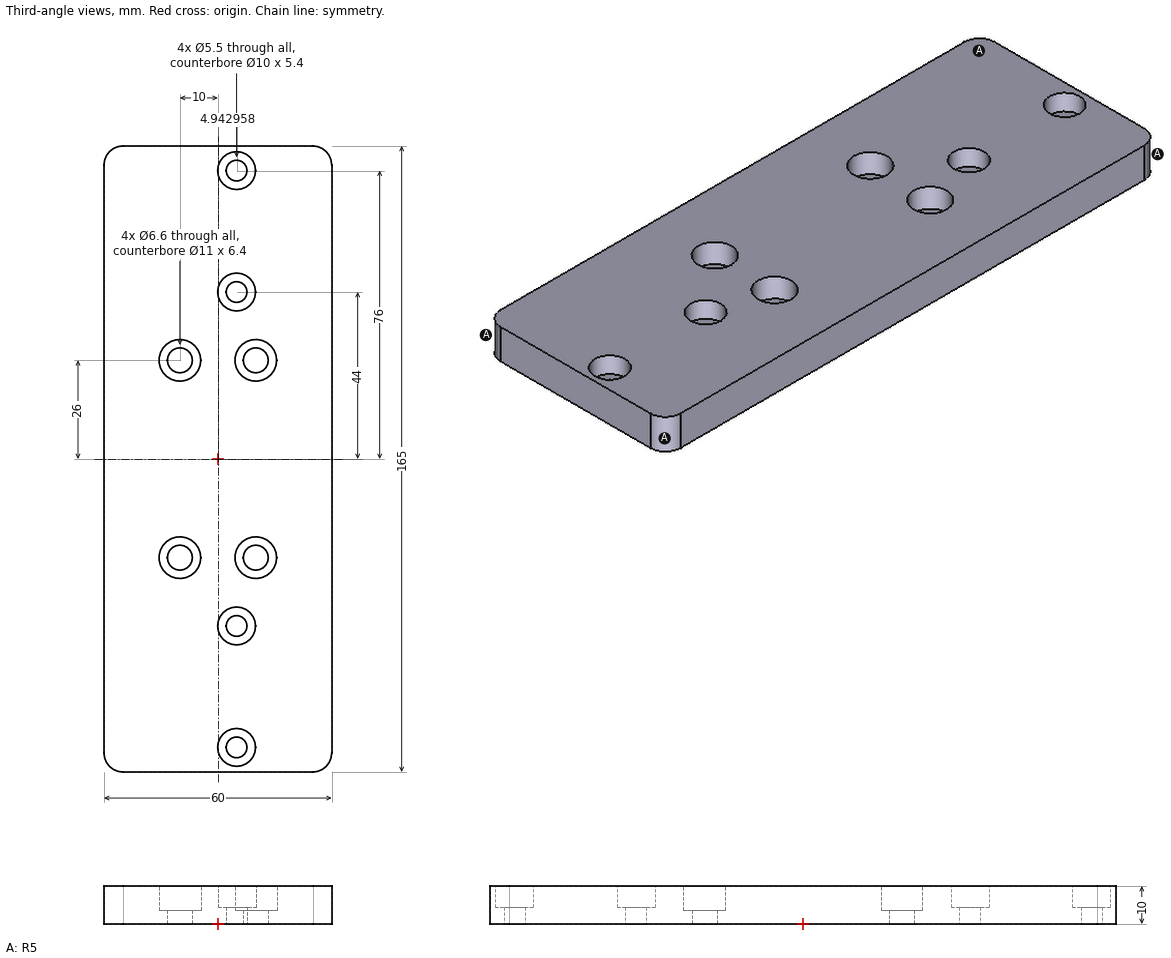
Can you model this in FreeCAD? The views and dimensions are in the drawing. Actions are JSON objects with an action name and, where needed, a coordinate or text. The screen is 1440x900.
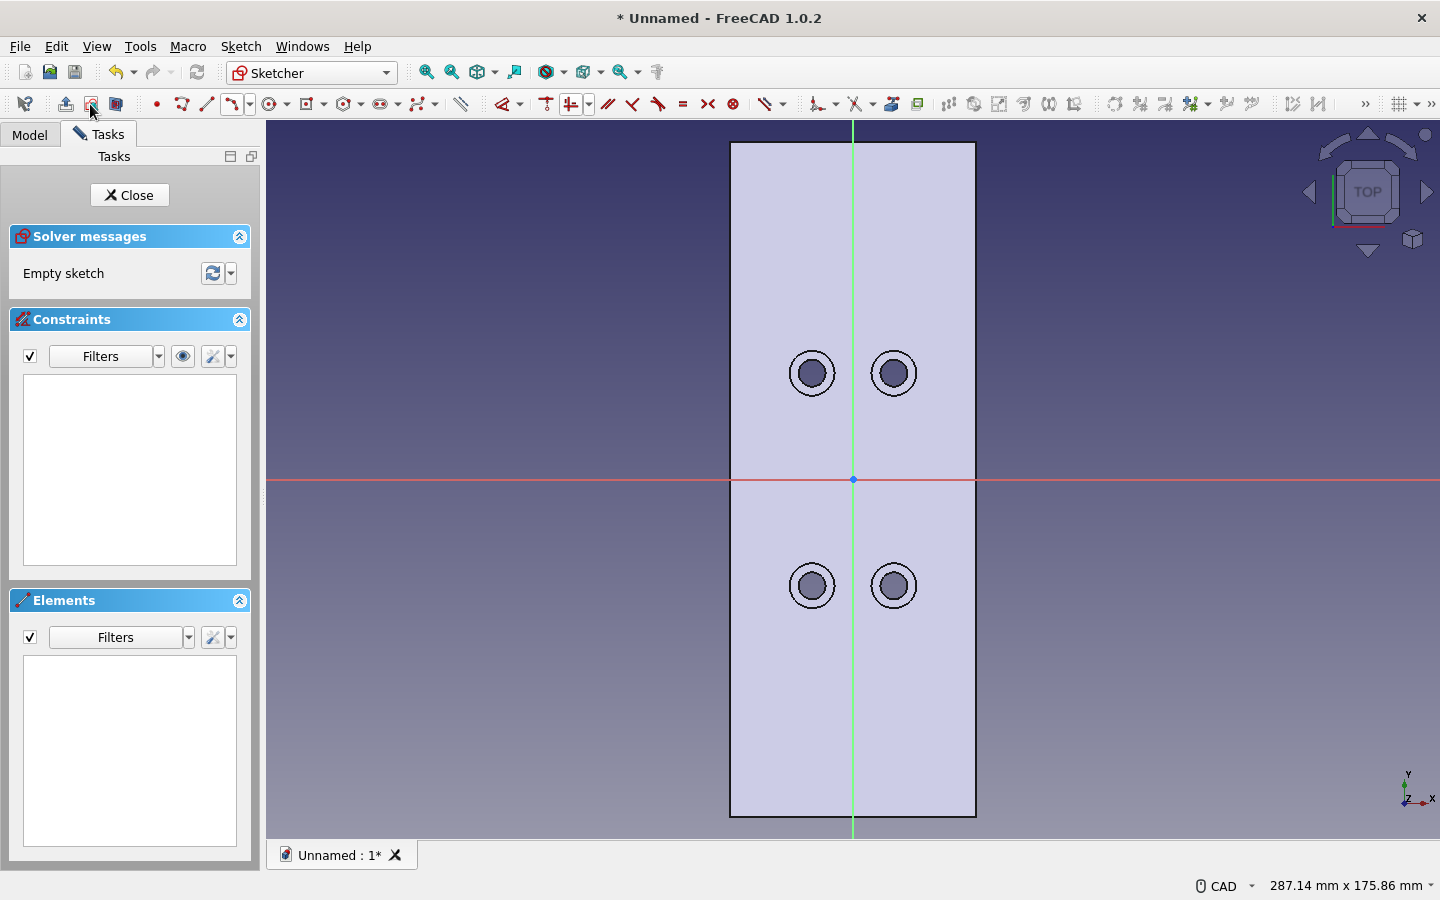
{"action": "scroll", "coordinate": [613, 480], "scroll_direction": "down", "scroll_amount": 2}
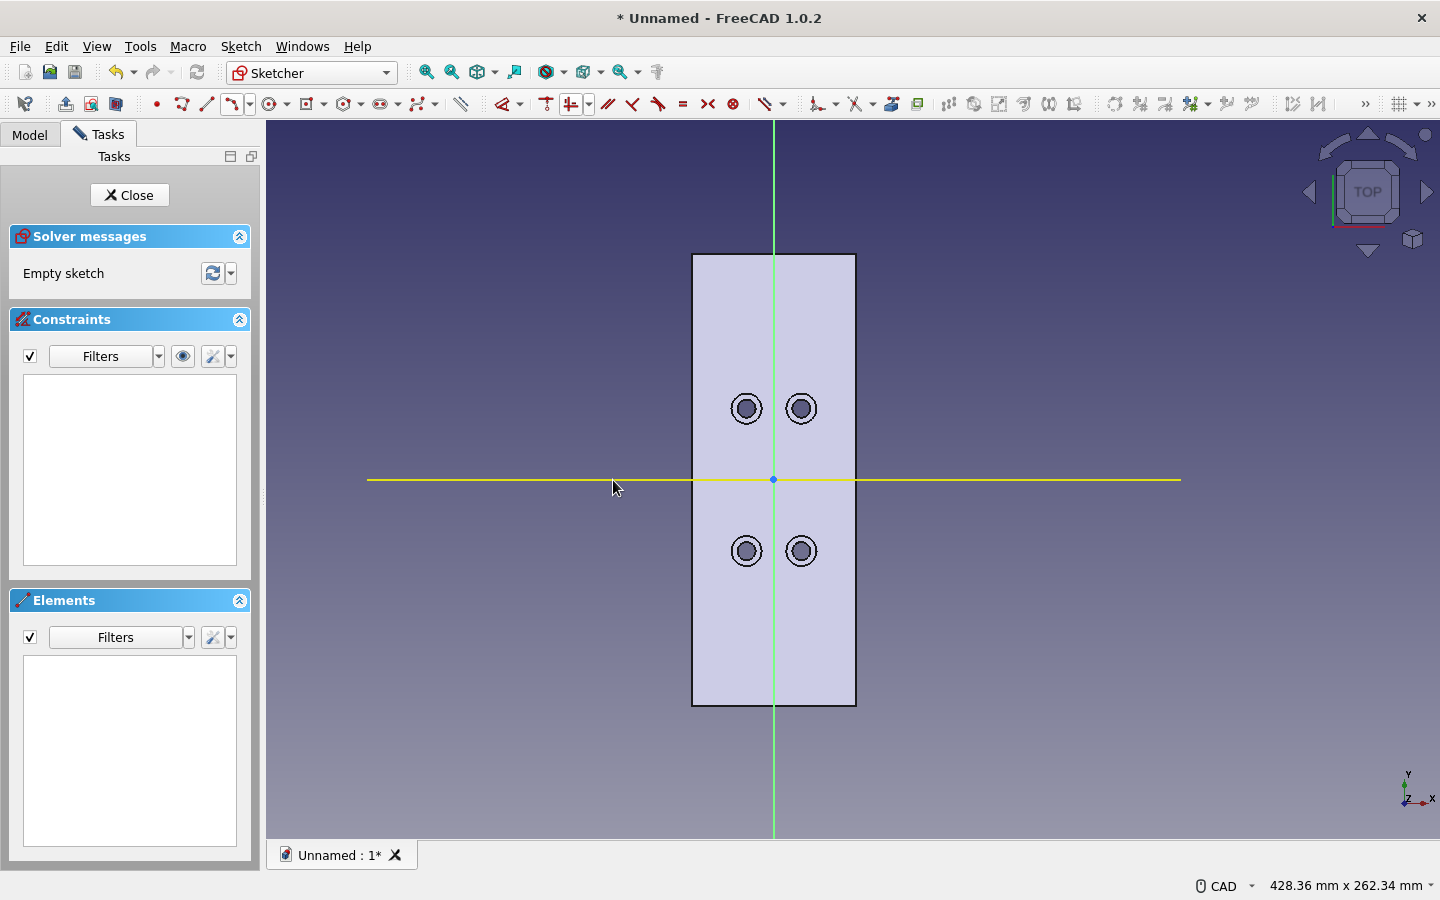
{"action": "key", "text": "g c"}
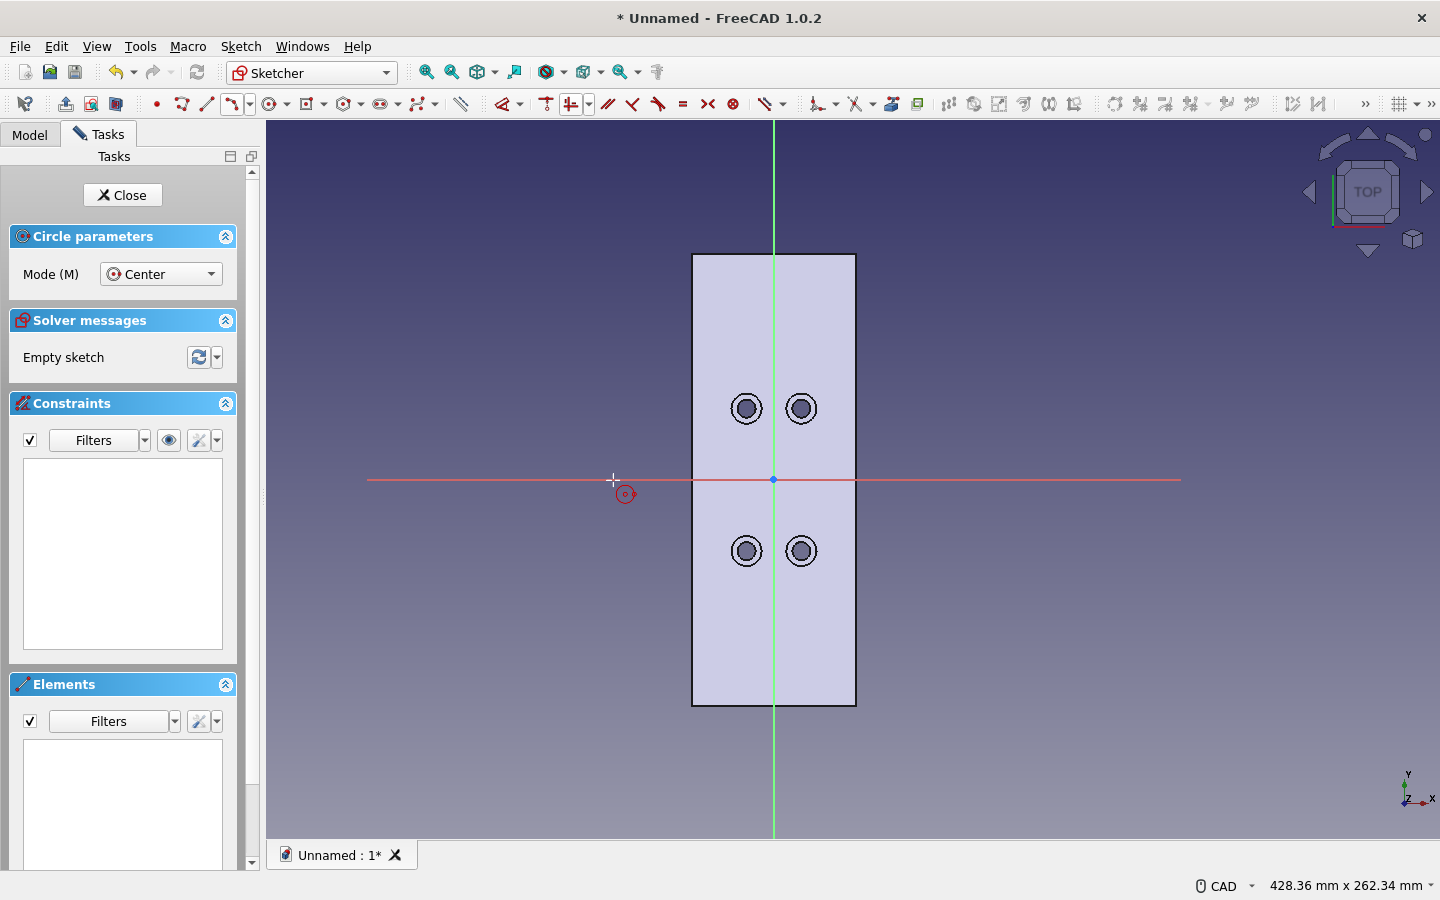
{"action": "scroll", "coordinate": [788, 272], "scroll_direction": "up", "scroll_amount": 6}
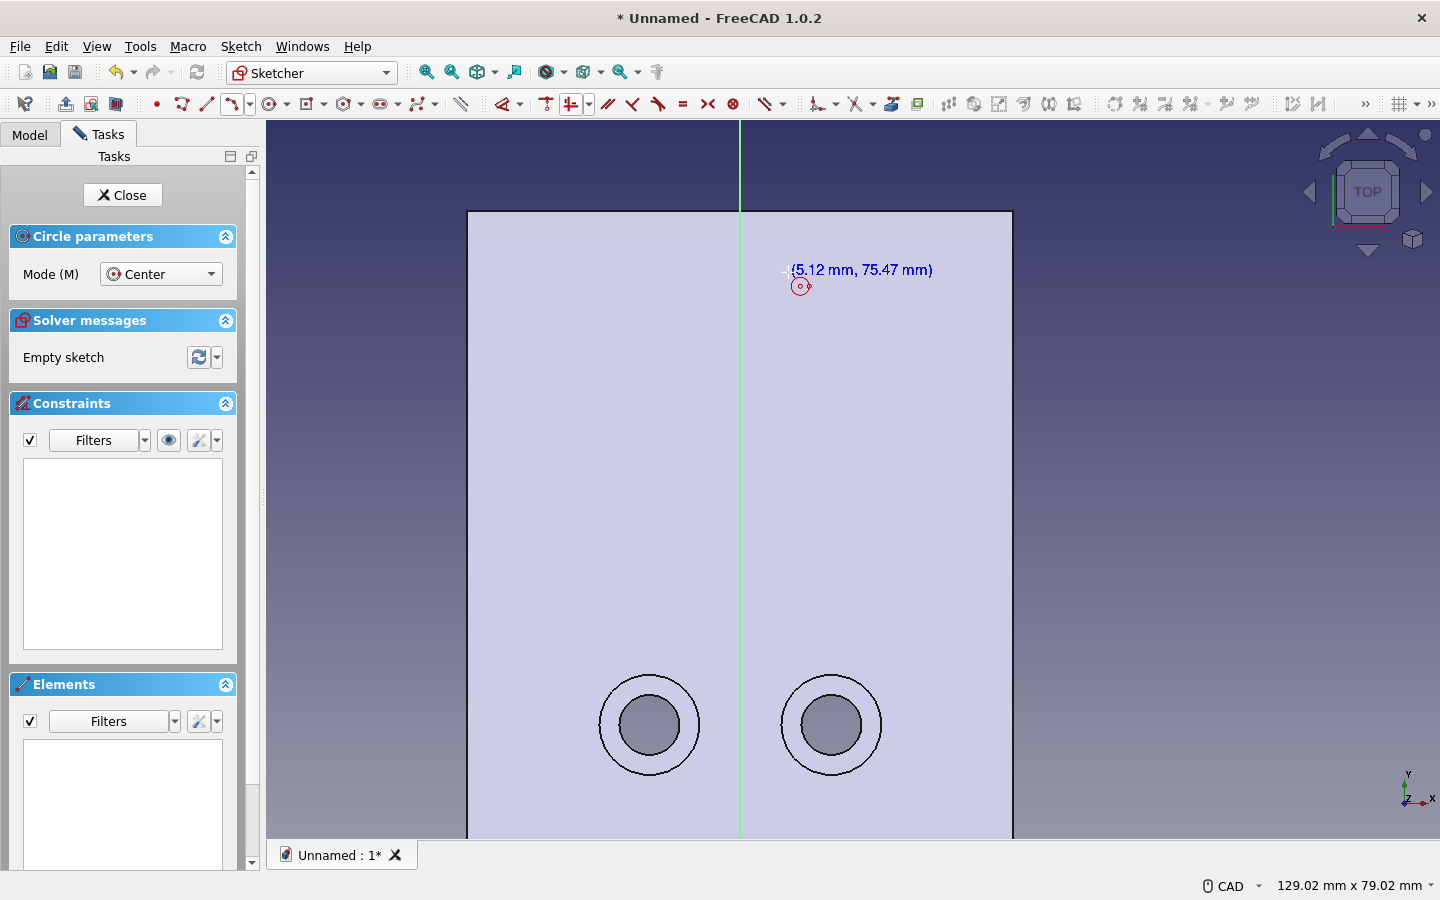
{"action": "left_click", "coordinate": [785, 270]}
{"action": "left_click", "coordinate": [803, 252]}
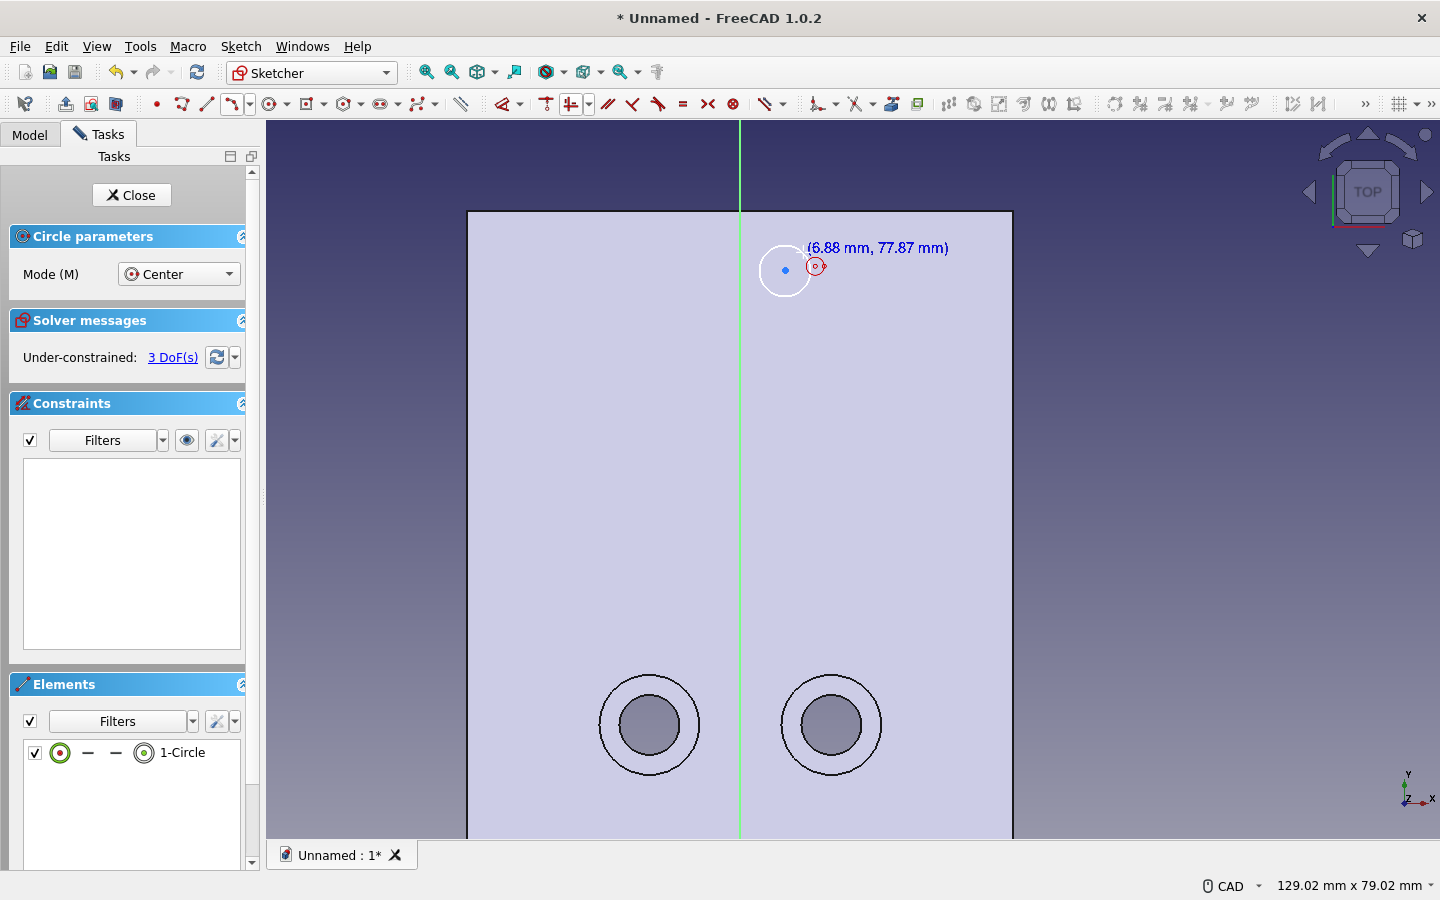
{"action": "left_click", "coordinate": [785, 561]}
{"action": "left_click", "coordinate": [803, 543]}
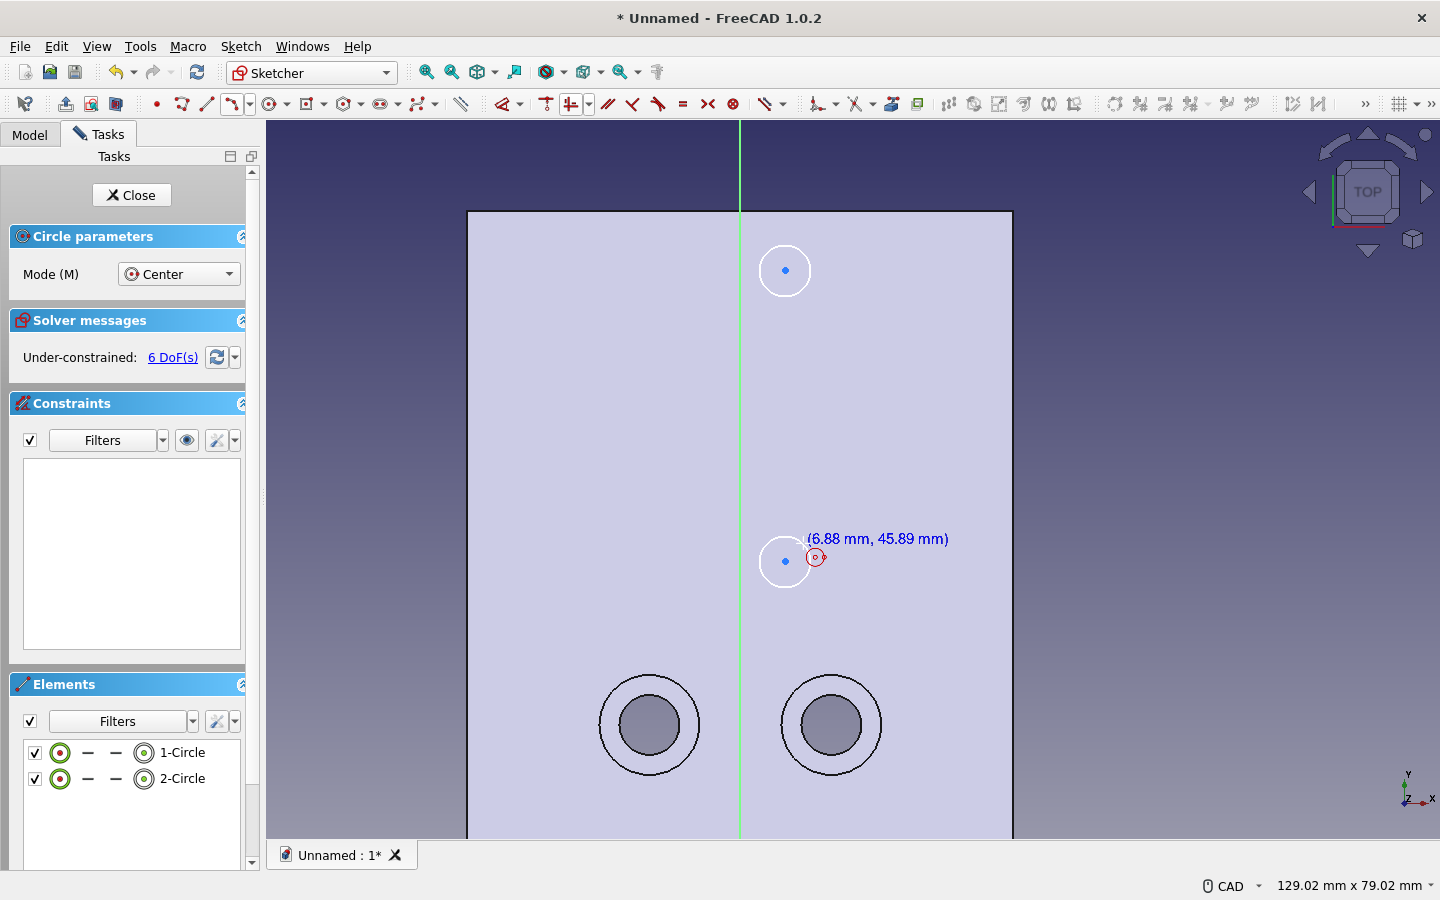
{"action": "scroll", "coordinate": [788, 272], "scroll_direction": "down", "scroll_amount": 6}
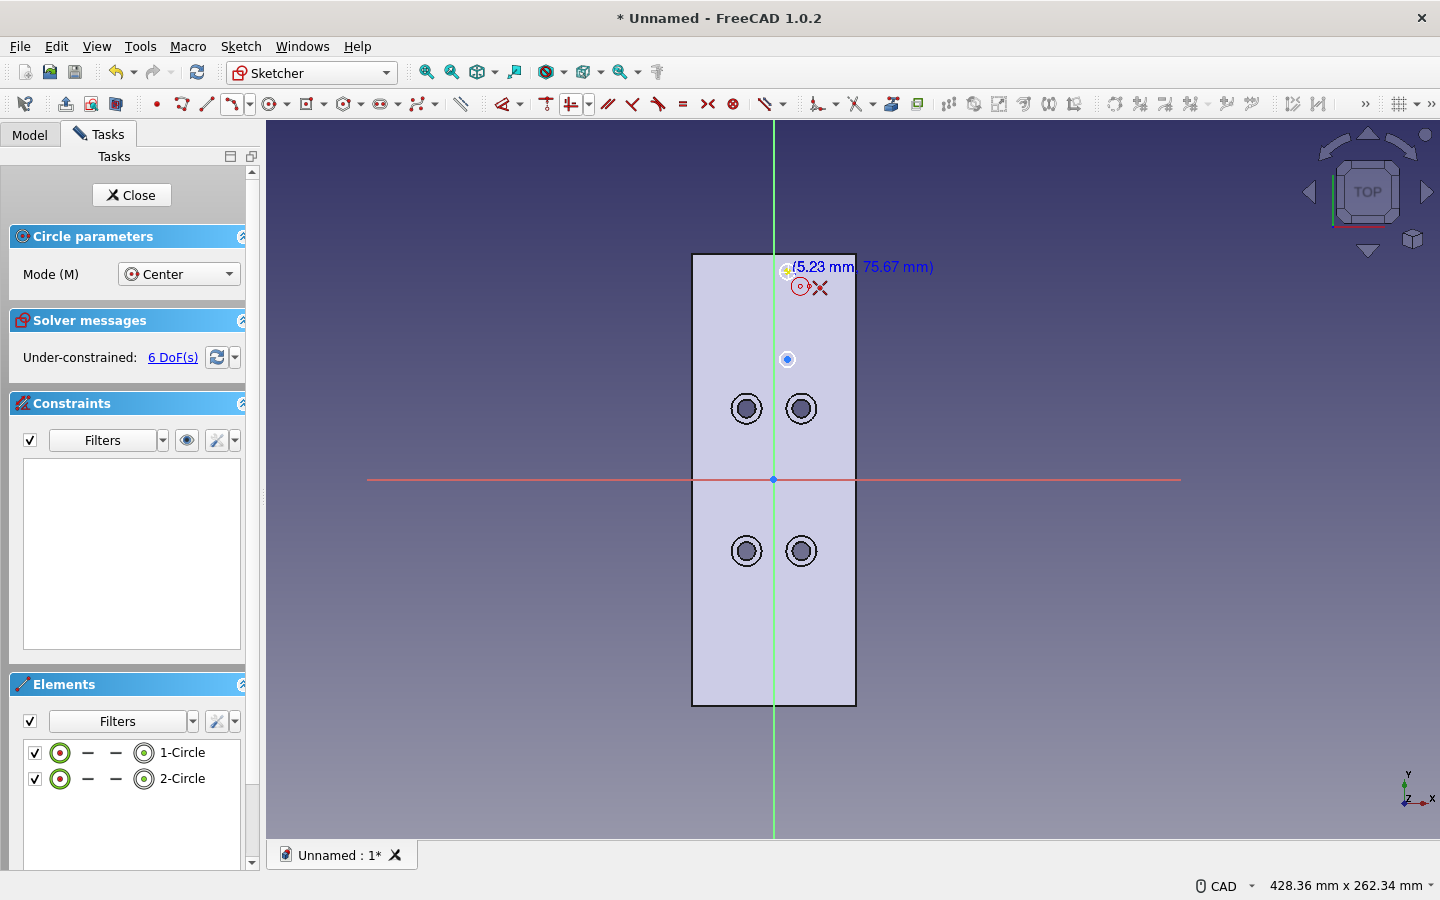
{"action": "scroll", "coordinate": [788, 600], "scroll_direction": "up", "scroll_amount": 6}